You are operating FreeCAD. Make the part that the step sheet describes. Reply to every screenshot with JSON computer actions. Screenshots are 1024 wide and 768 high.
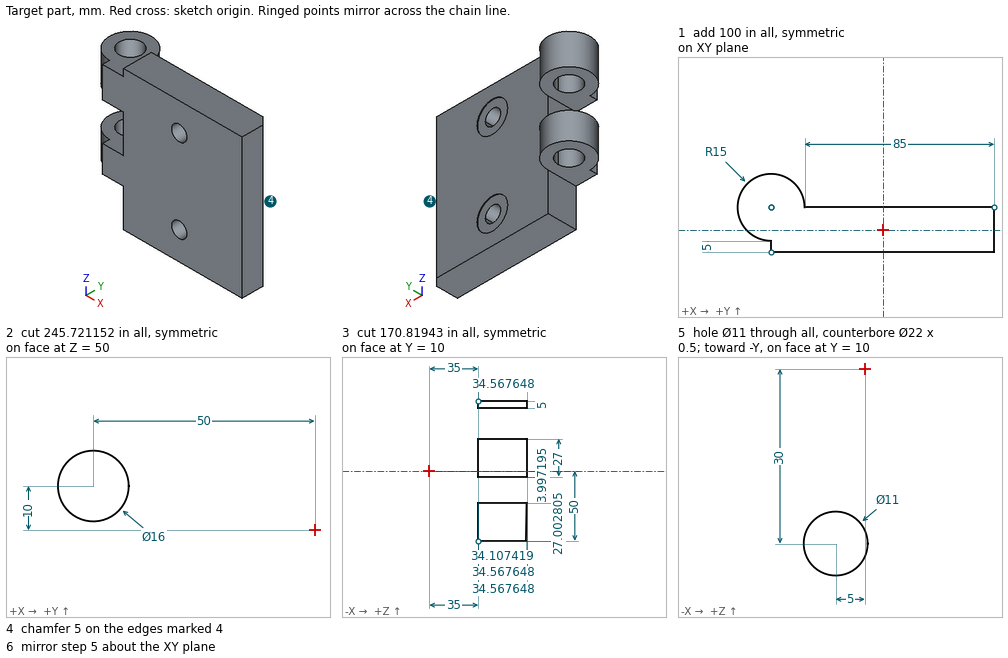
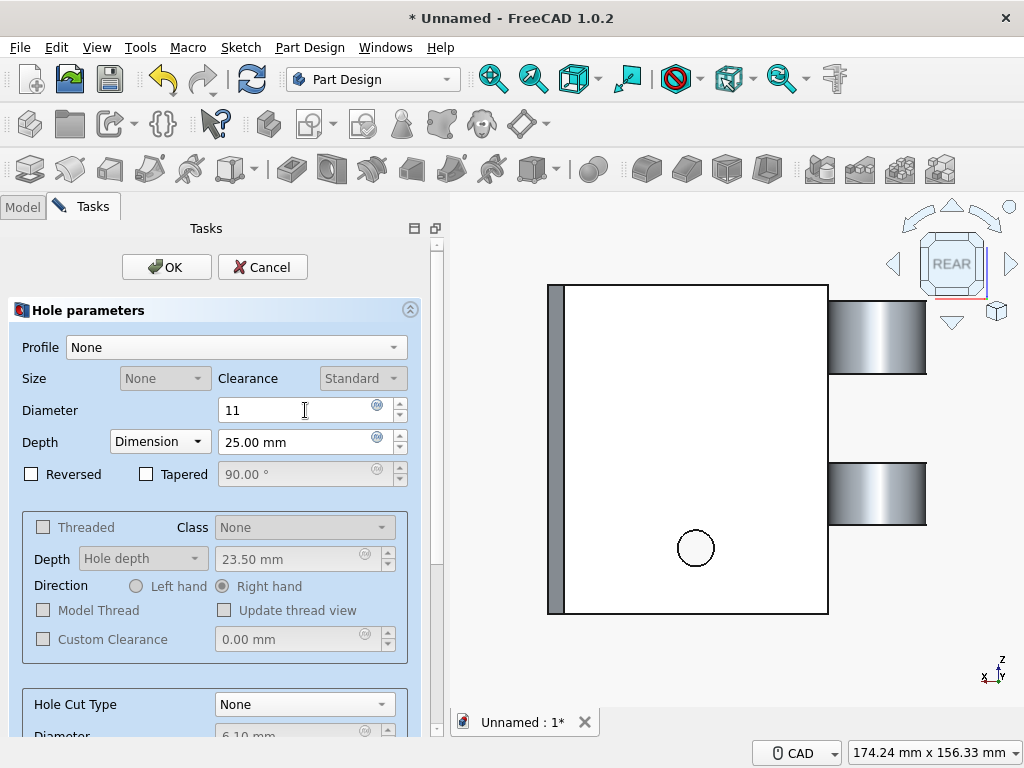
{"action": "left_click", "coordinate": [161, 442]}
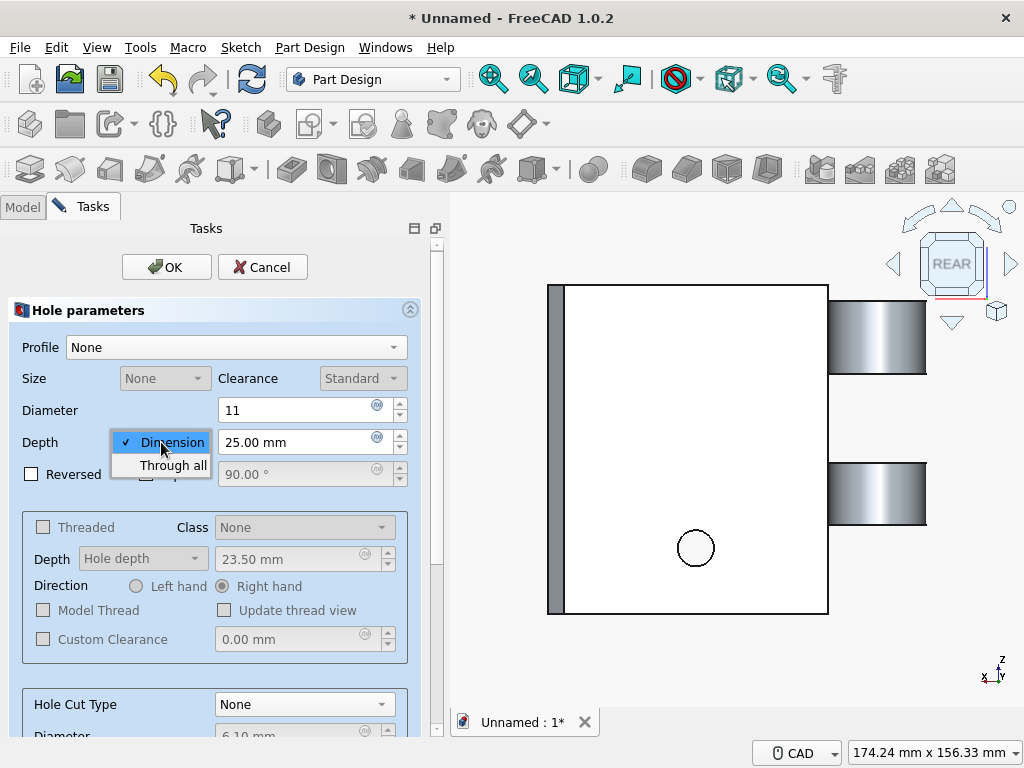
{"action": "left_click", "coordinate": [160, 466]}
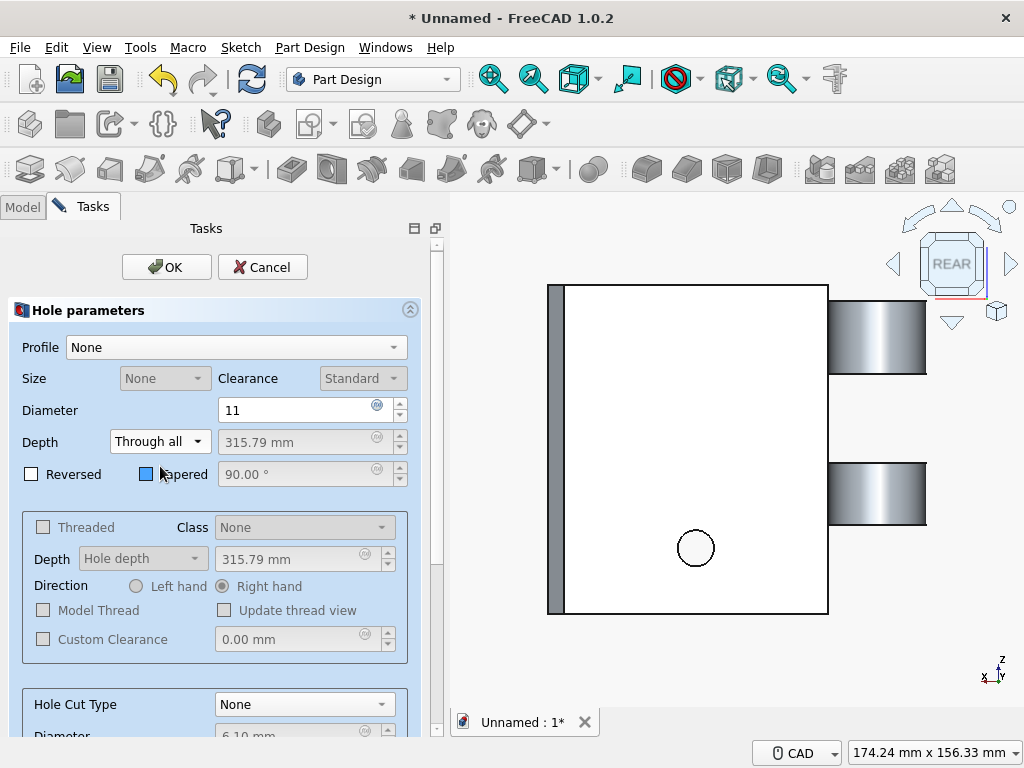
{"action": "left_click", "coordinate": [306, 704]}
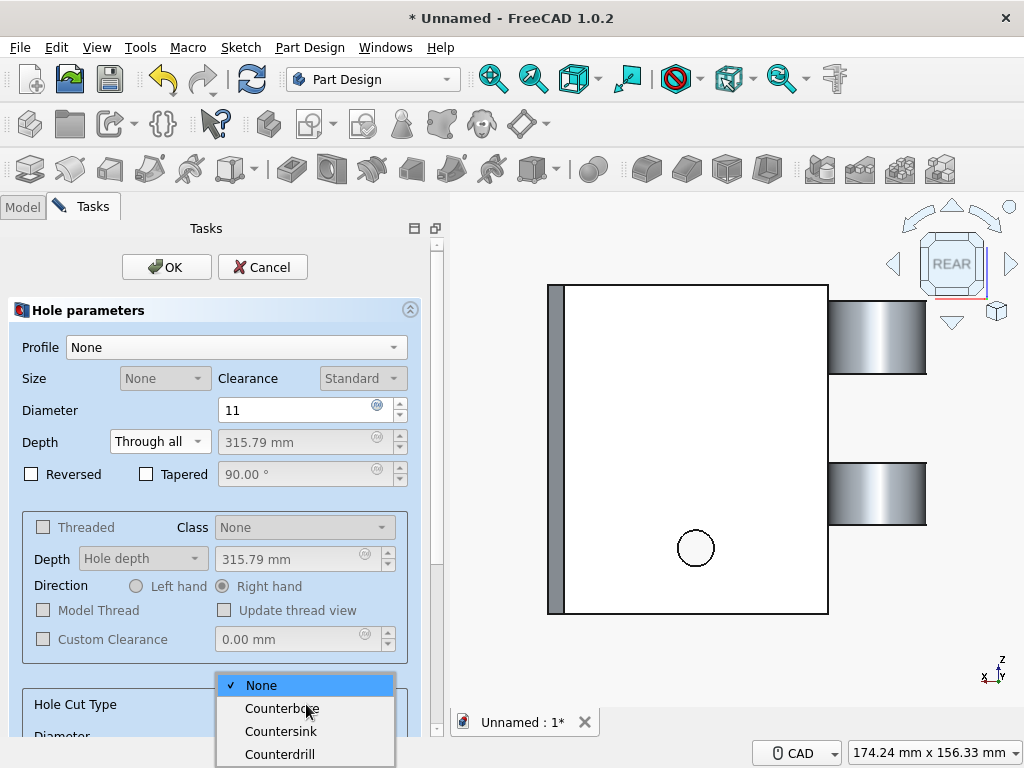
{"action": "left_click", "coordinate": [304, 708]}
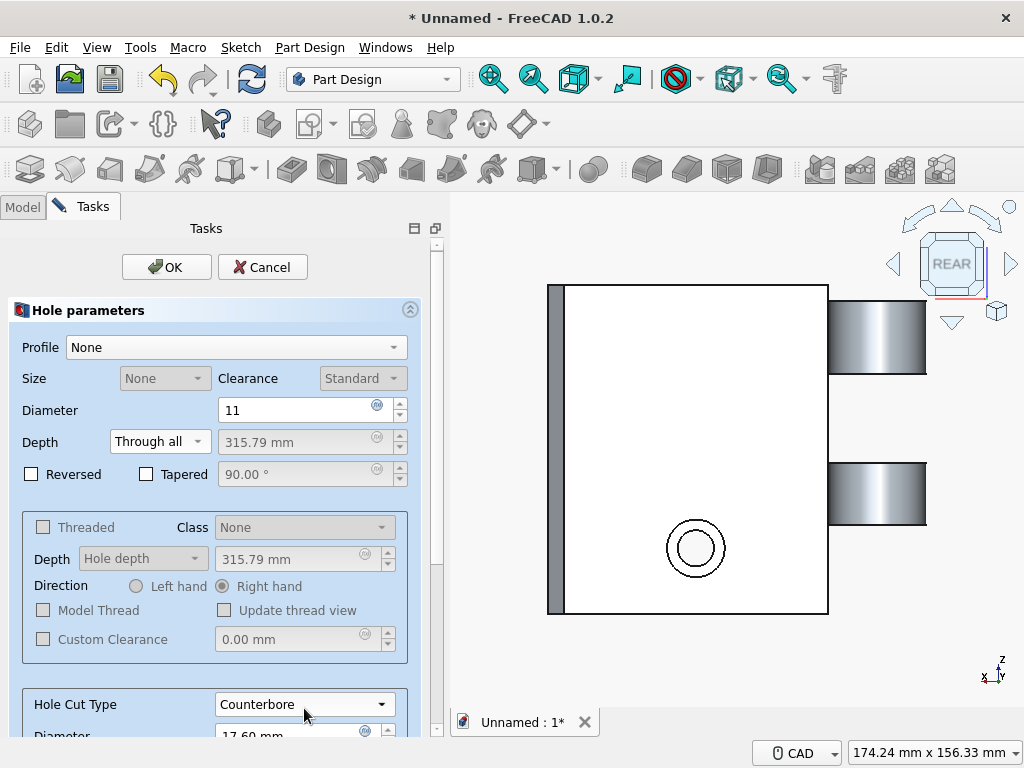
{"action": "scroll", "coordinate": [437, 487], "scroll_direction": "down", "scroll_amount": 2}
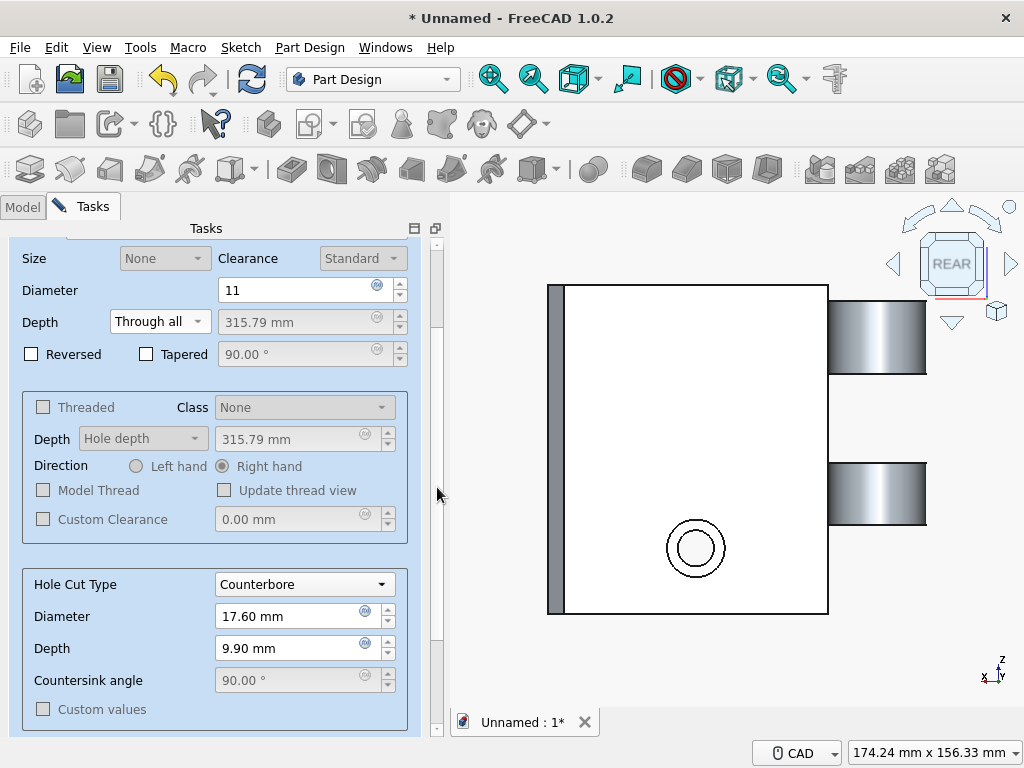
{"action": "triple_click", "coordinate": [298, 616]}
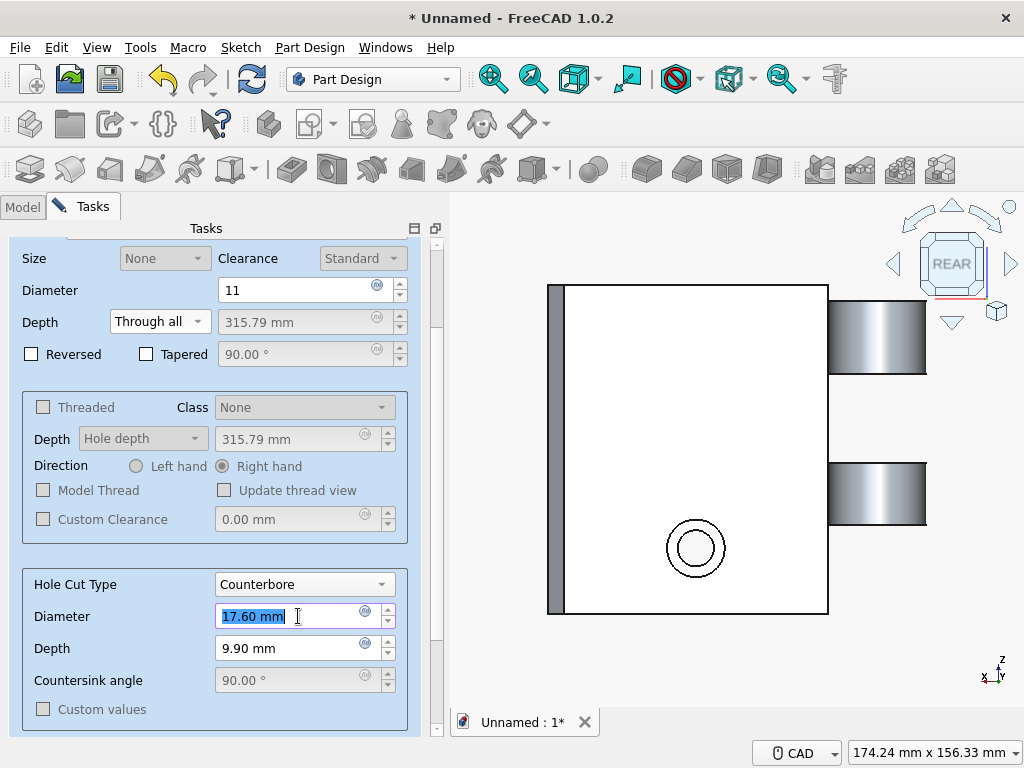
{"action": "type", "text": "22"}
{"action": "key", "text": "Tab"}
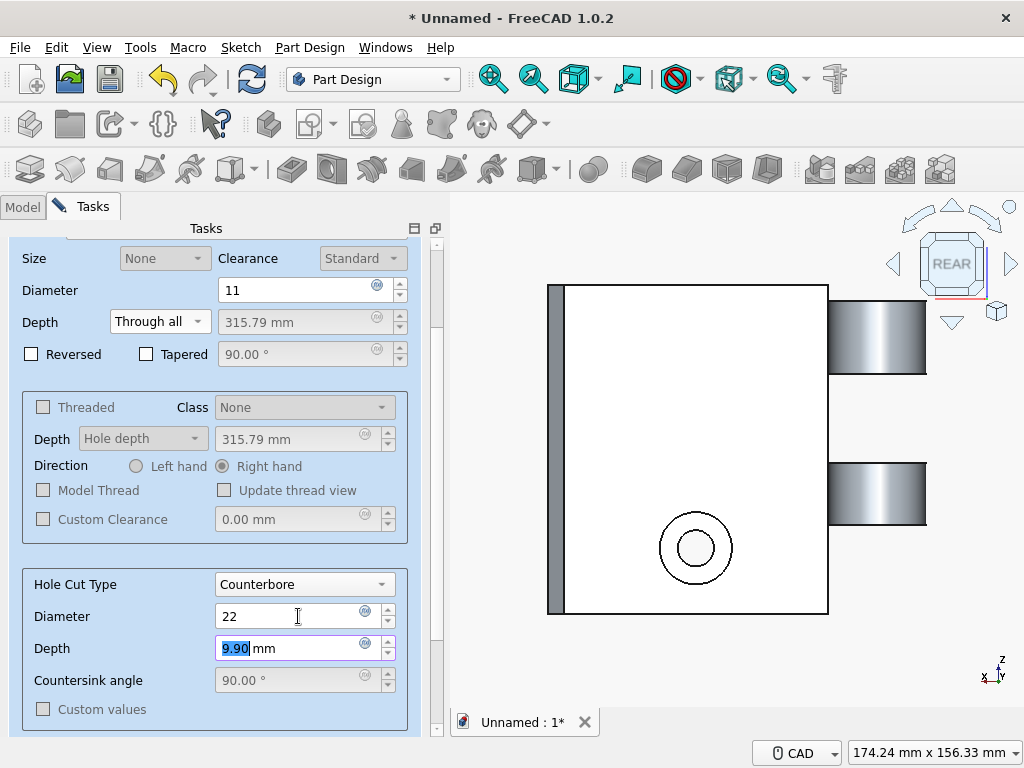
{"action": "type", "text": "0.5"}
{"action": "key", "text": "Tab"}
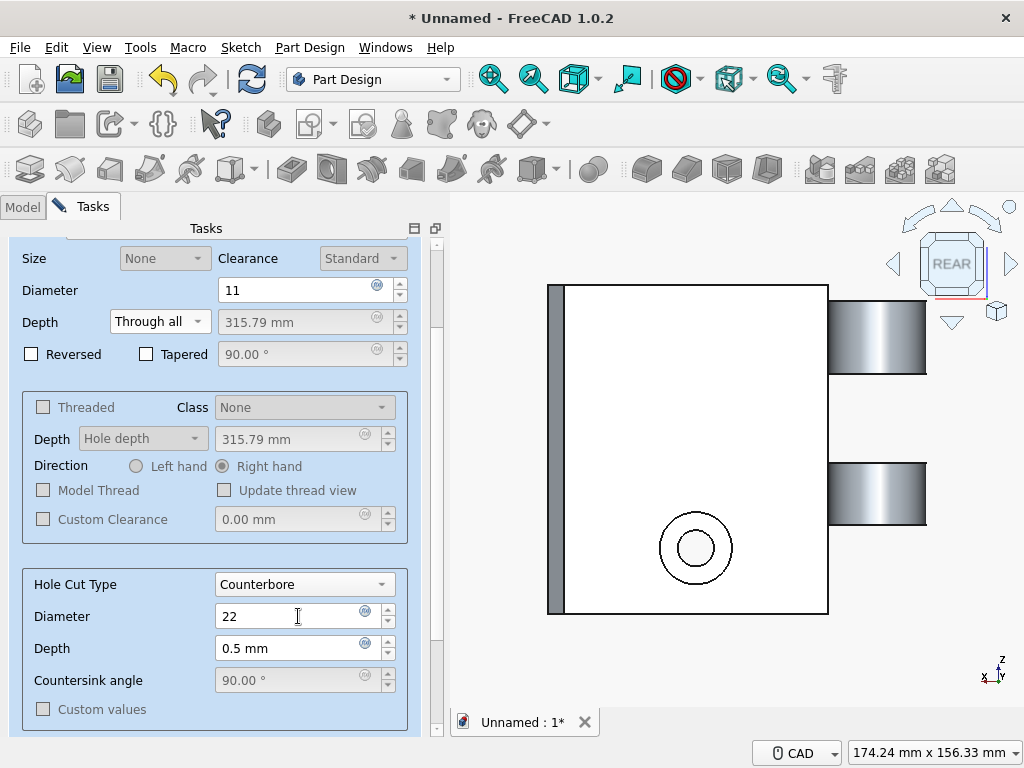
{"action": "scroll", "coordinate": [437, 487], "scroll_direction": "up", "scroll_amount": 3}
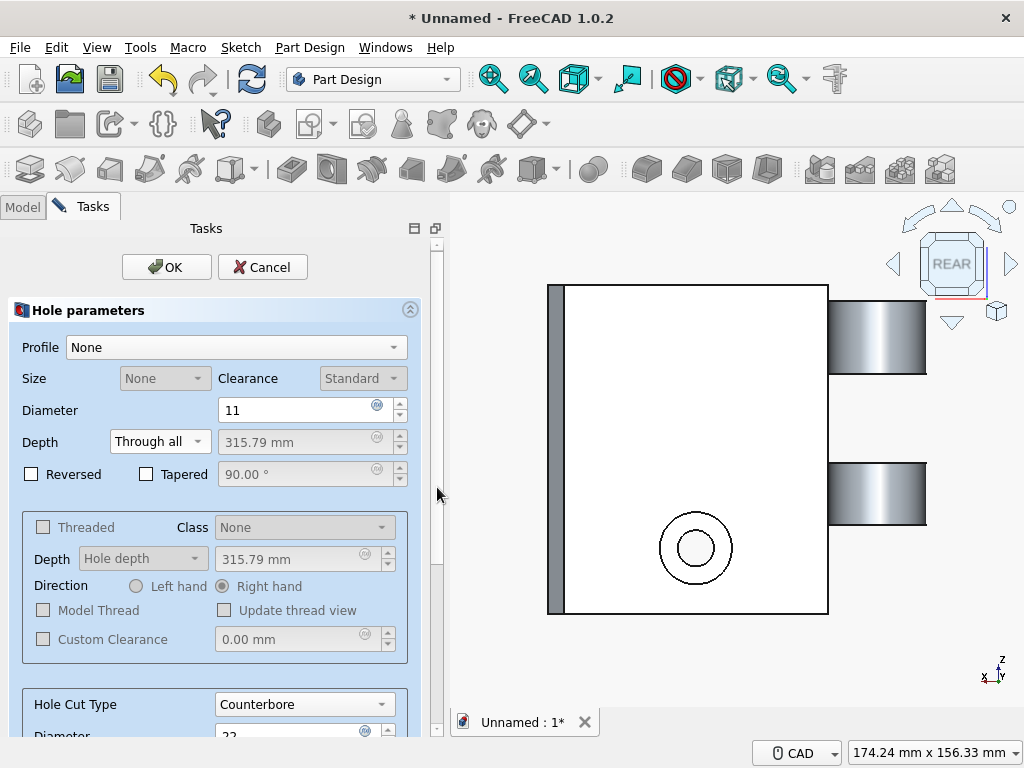
{"action": "left_click", "coordinate": [167, 267]}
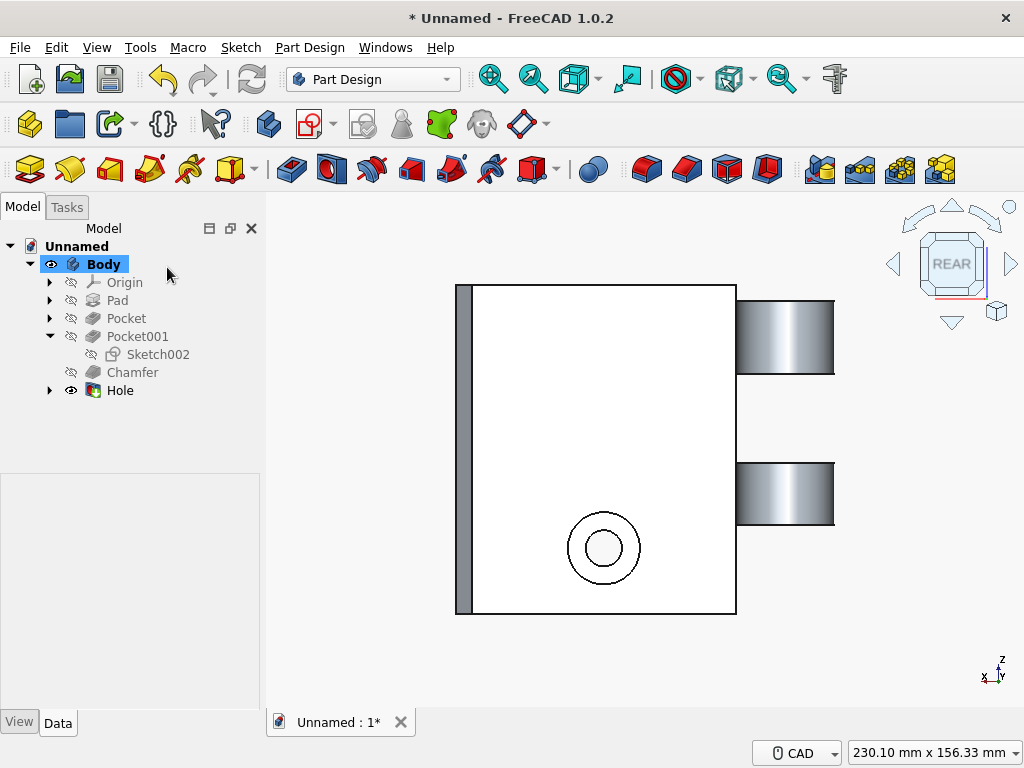
{"action": "left_click", "coordinate": [116, 390]}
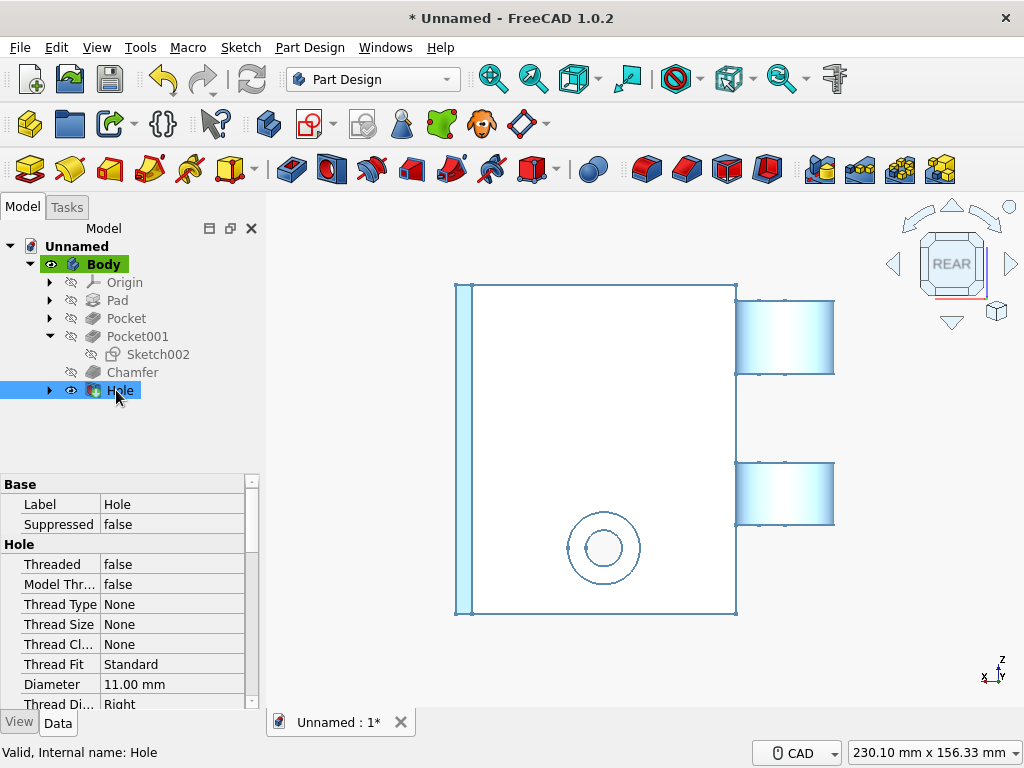
{"action": "left_click", "coordinate": [820, 170]}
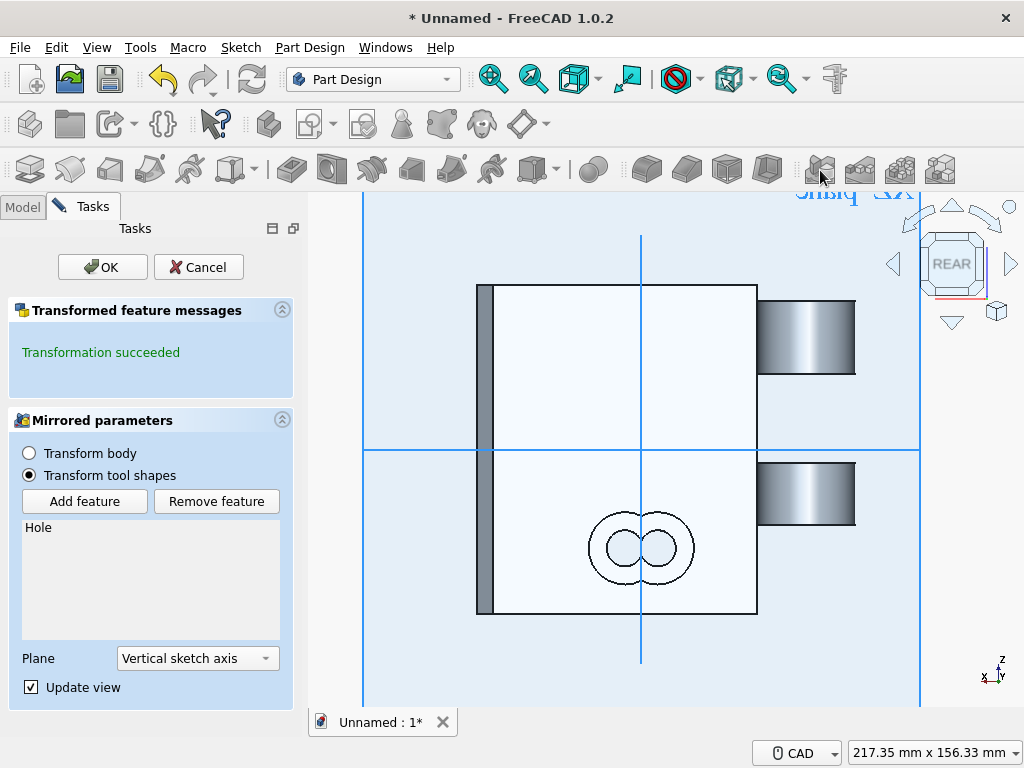
{"action": "left_click", "coordinate": [198, 658]}